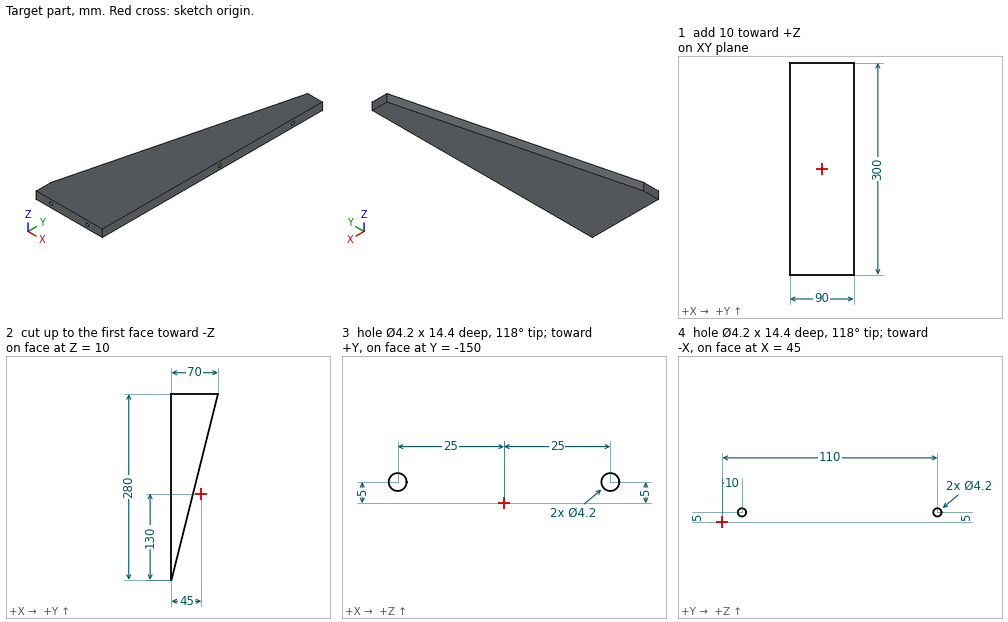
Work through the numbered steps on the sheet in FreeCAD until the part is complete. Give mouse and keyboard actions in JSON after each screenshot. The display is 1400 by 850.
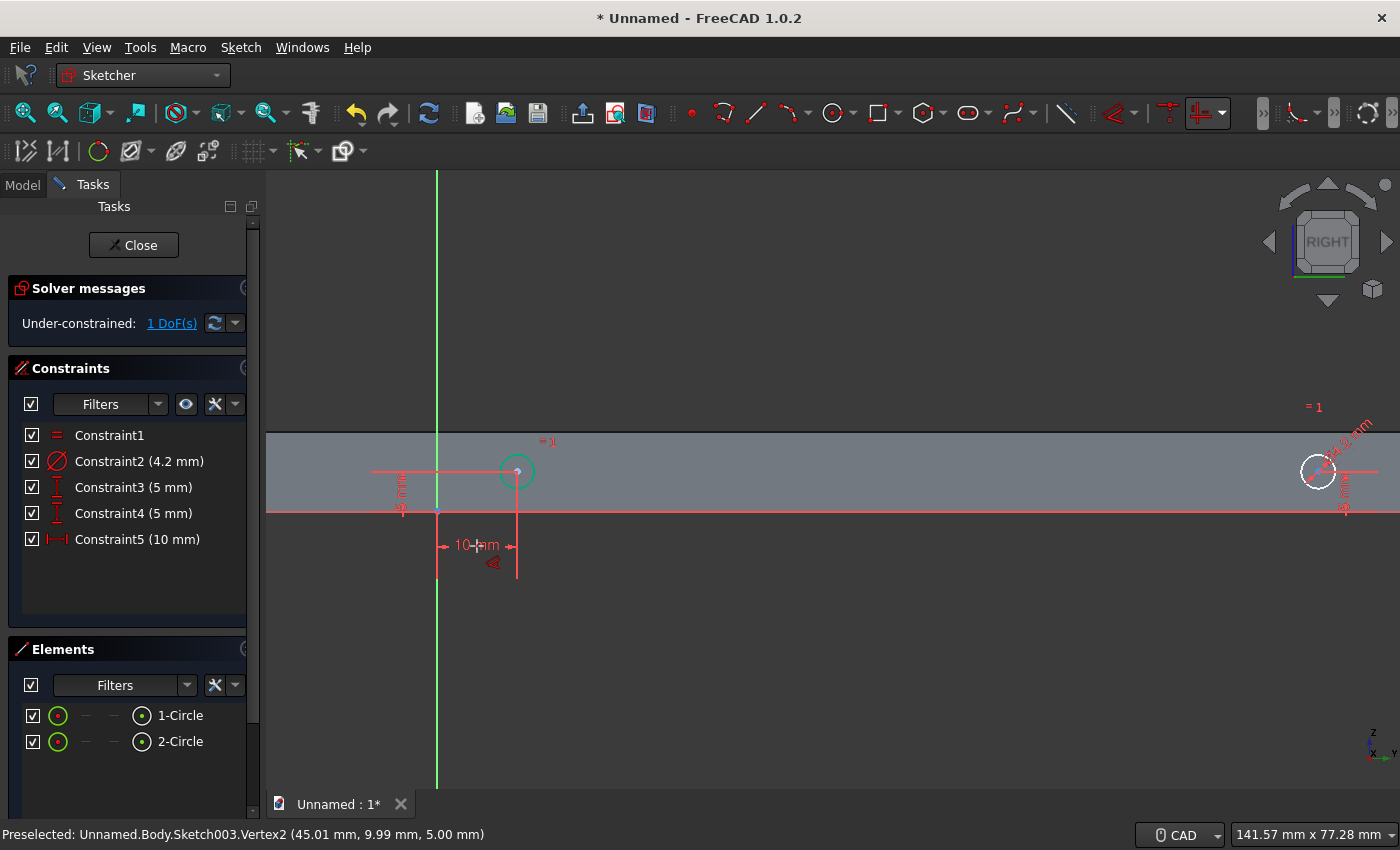
{"action": "scroll", "coordinate": [517, 472], "scroll_direction": "down", "scroll_amount": 2}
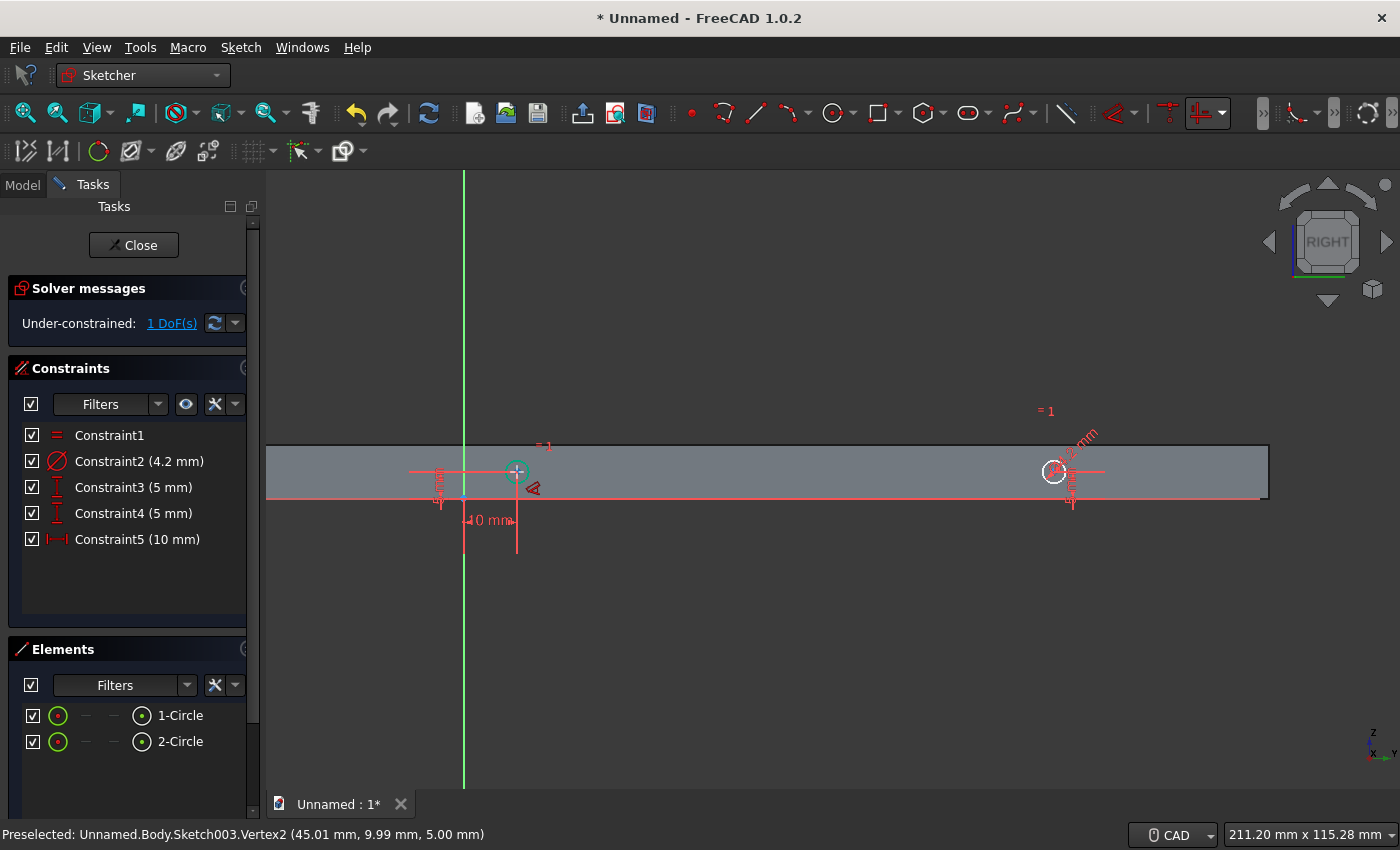
{"action": "left_click", "coordinate": [1054, 472]}
{"action": "left_click", "coordinate": [759, 533]}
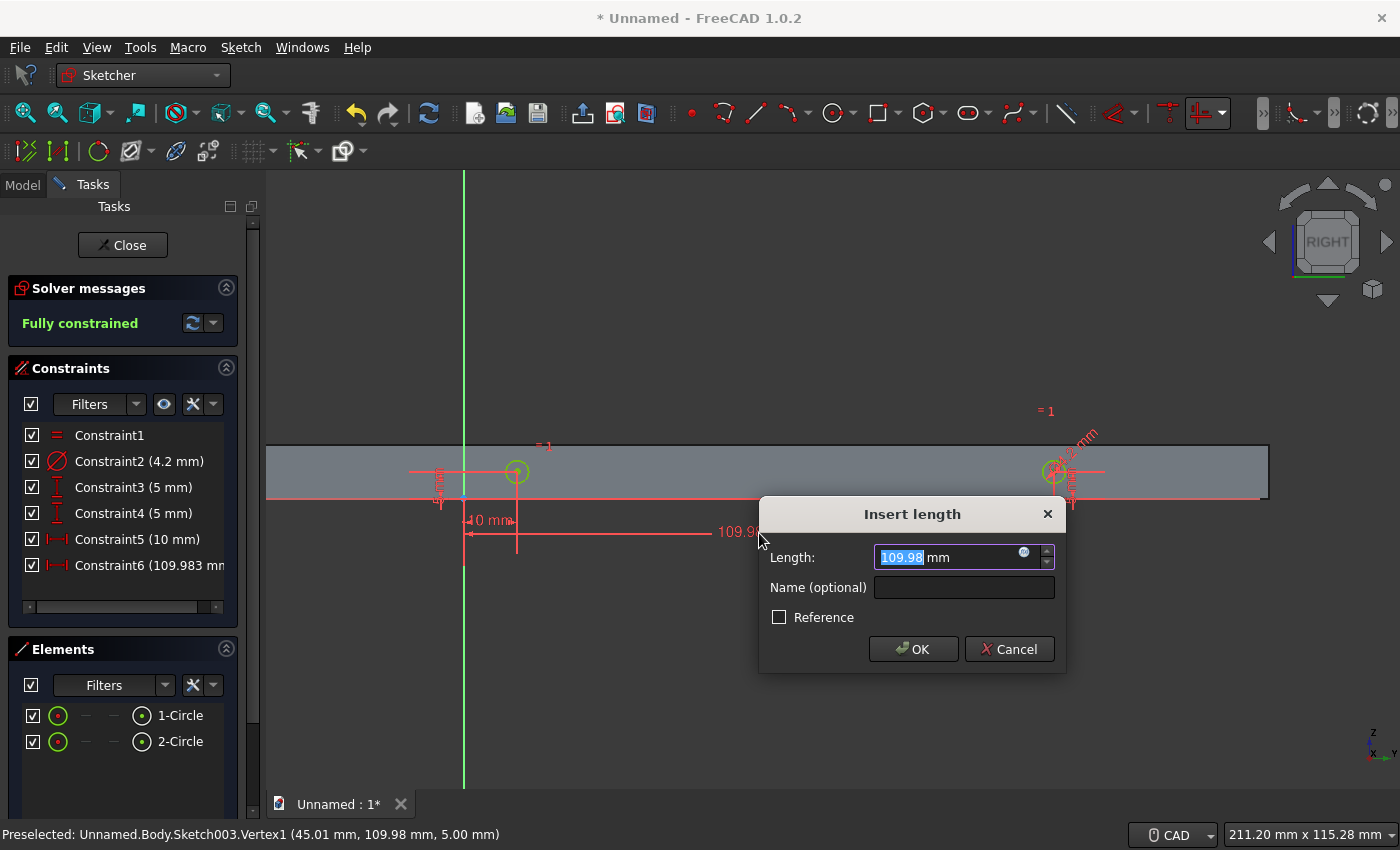
{"action": "type", "text": "110"}
{"action": "key", "text": "Return"}
{"action": "key", "text": "Escape"}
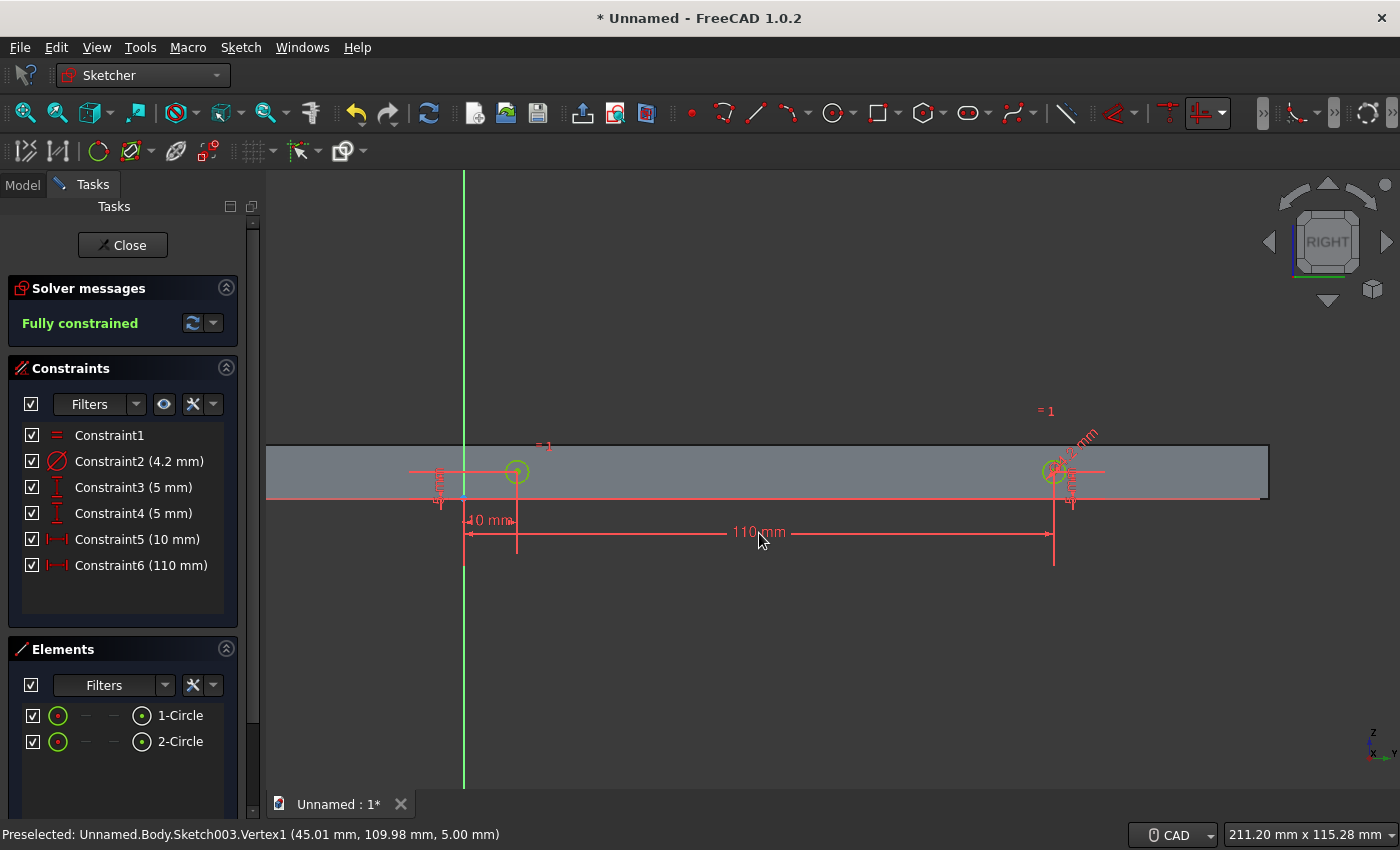
{"action": "left_click", "coordinate": [123, 245]}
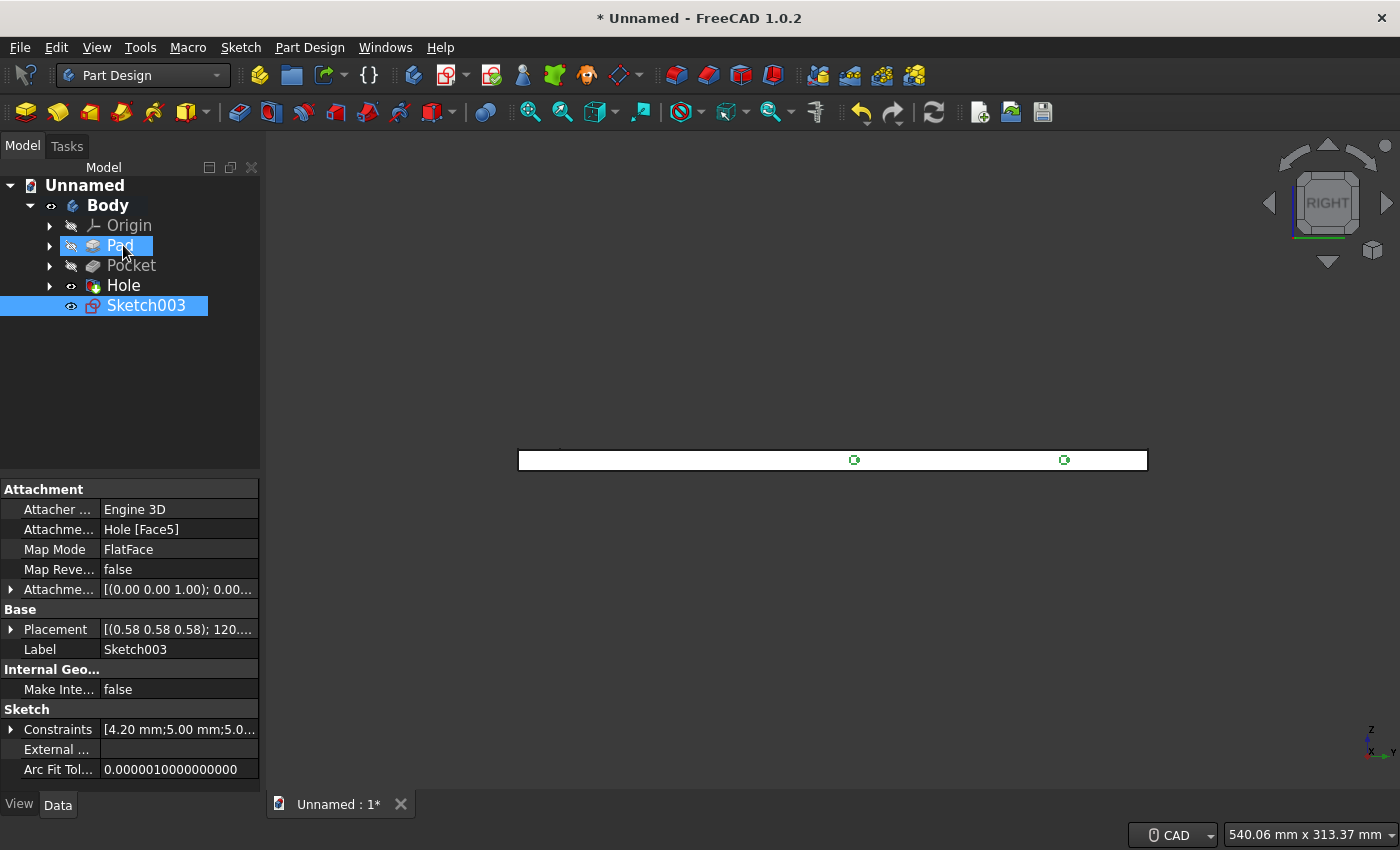
{"action": "left_click", "coordinate": [272, 112]}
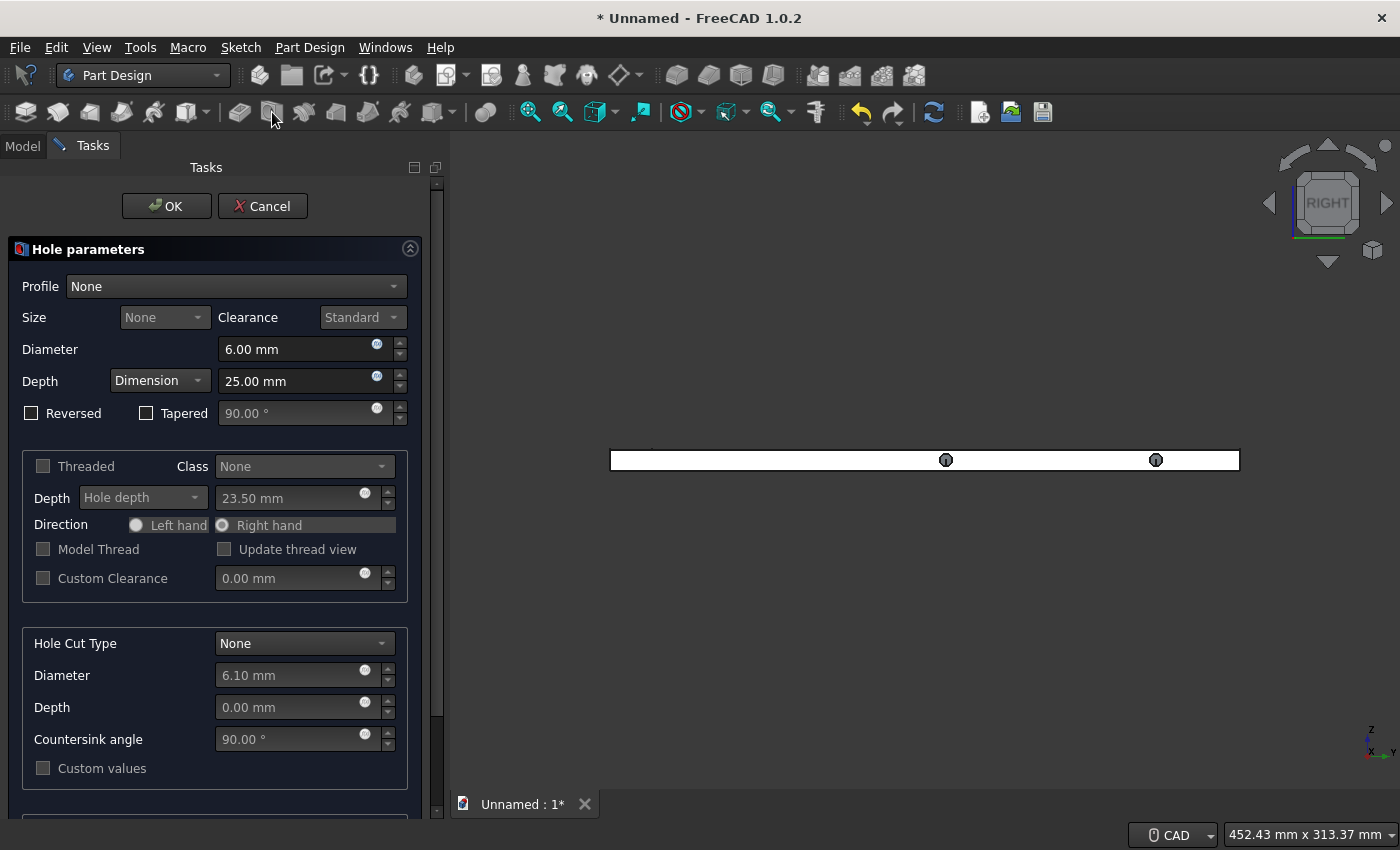
{"action": "triple_click", "coordinate": [305, 349]}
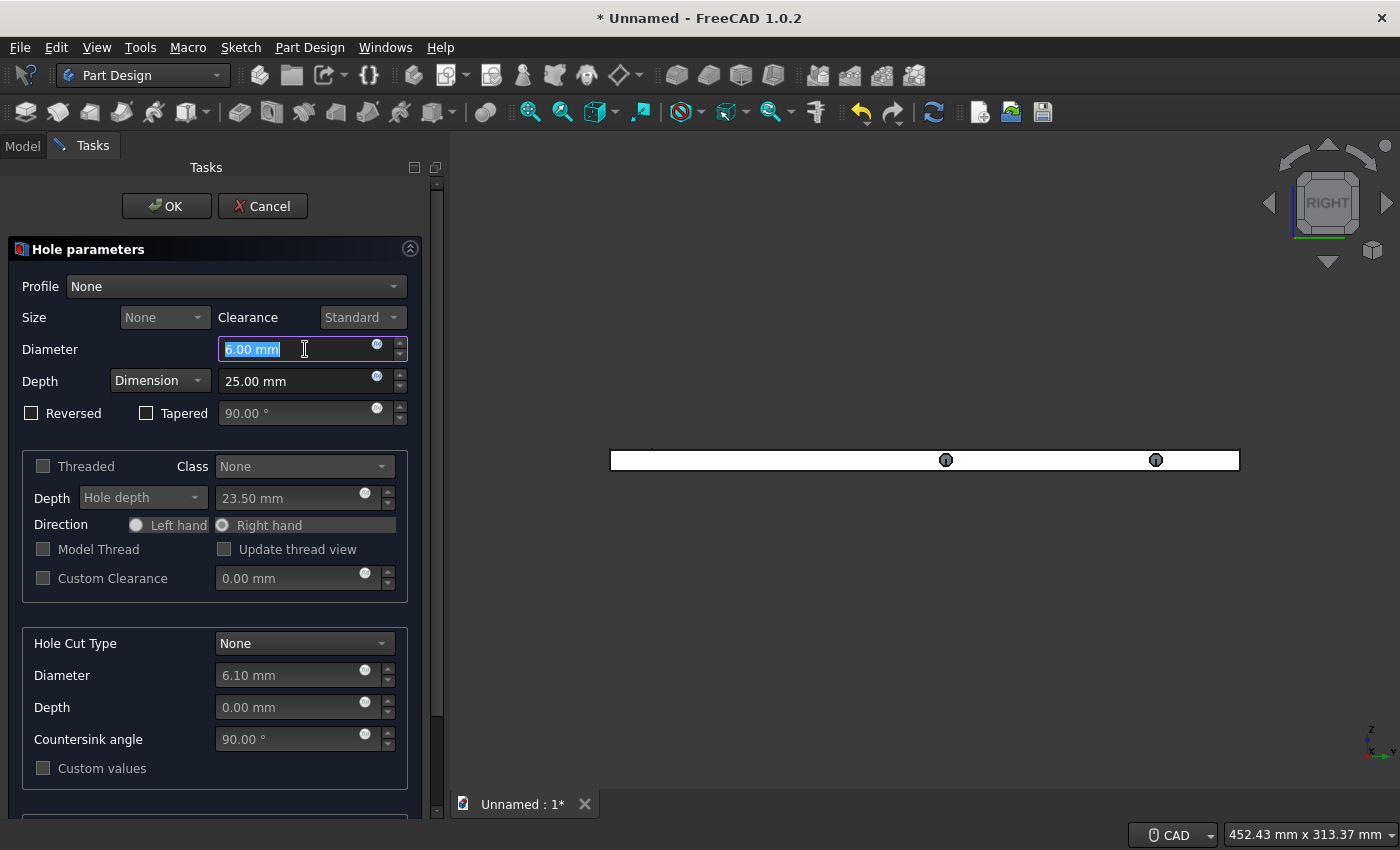
{"action": "type", "text": "4.2"}
{"action": "key", "text": "Tab"}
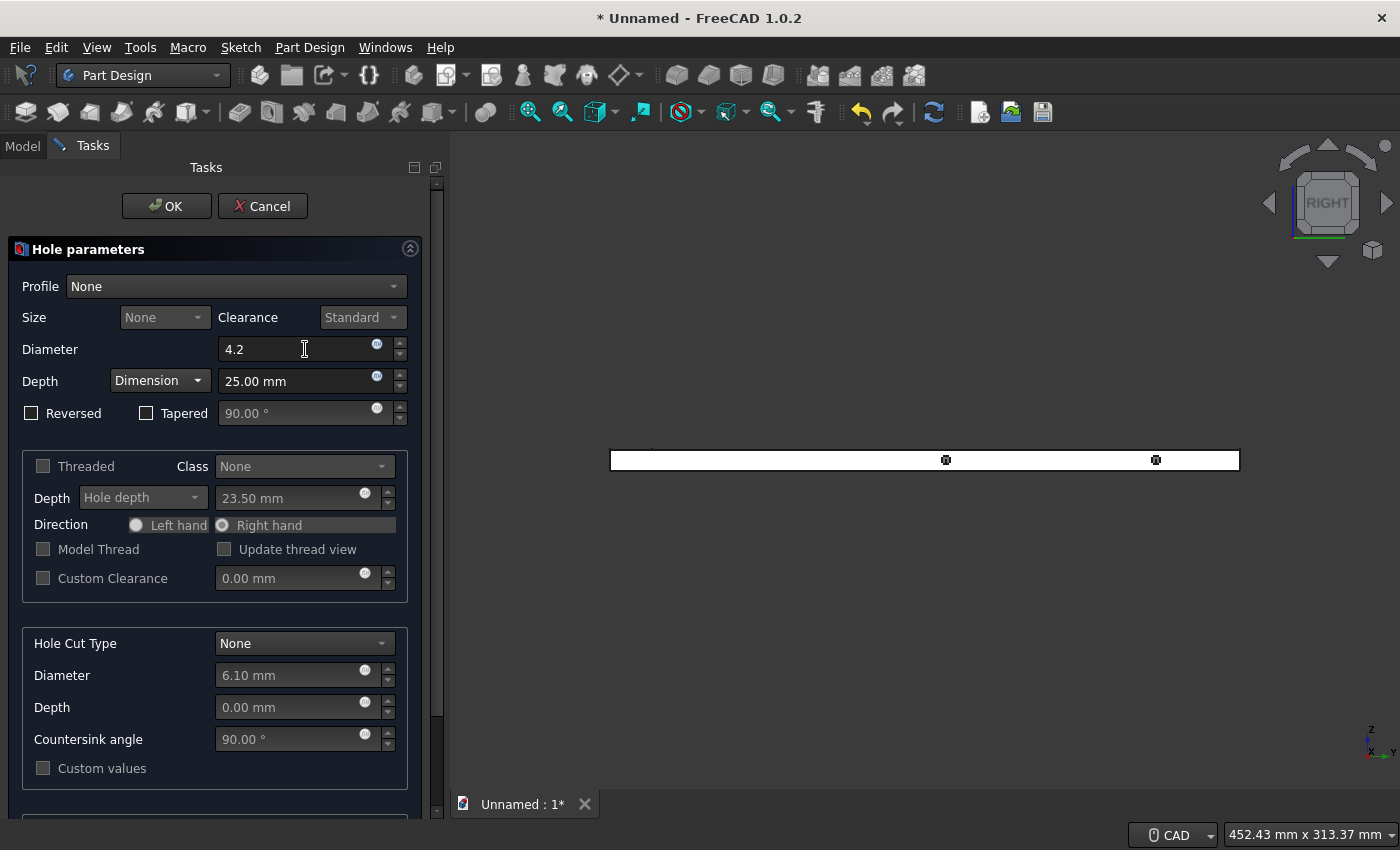
{"action": "triple_click", "coordinate": [305, 381]}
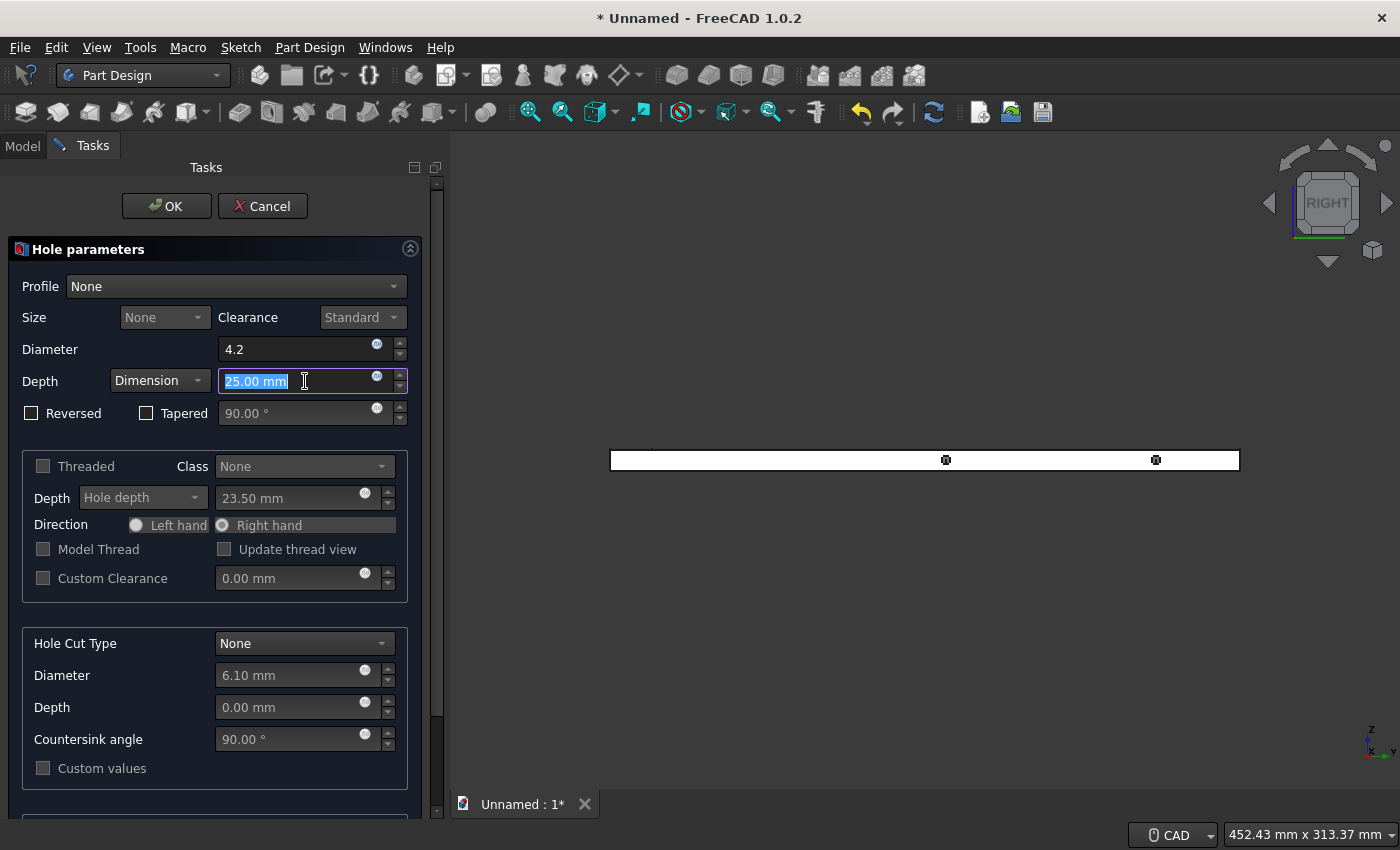
{"action": "type", "text": "14.4"}
{"action": "key", "text": "Tab"}